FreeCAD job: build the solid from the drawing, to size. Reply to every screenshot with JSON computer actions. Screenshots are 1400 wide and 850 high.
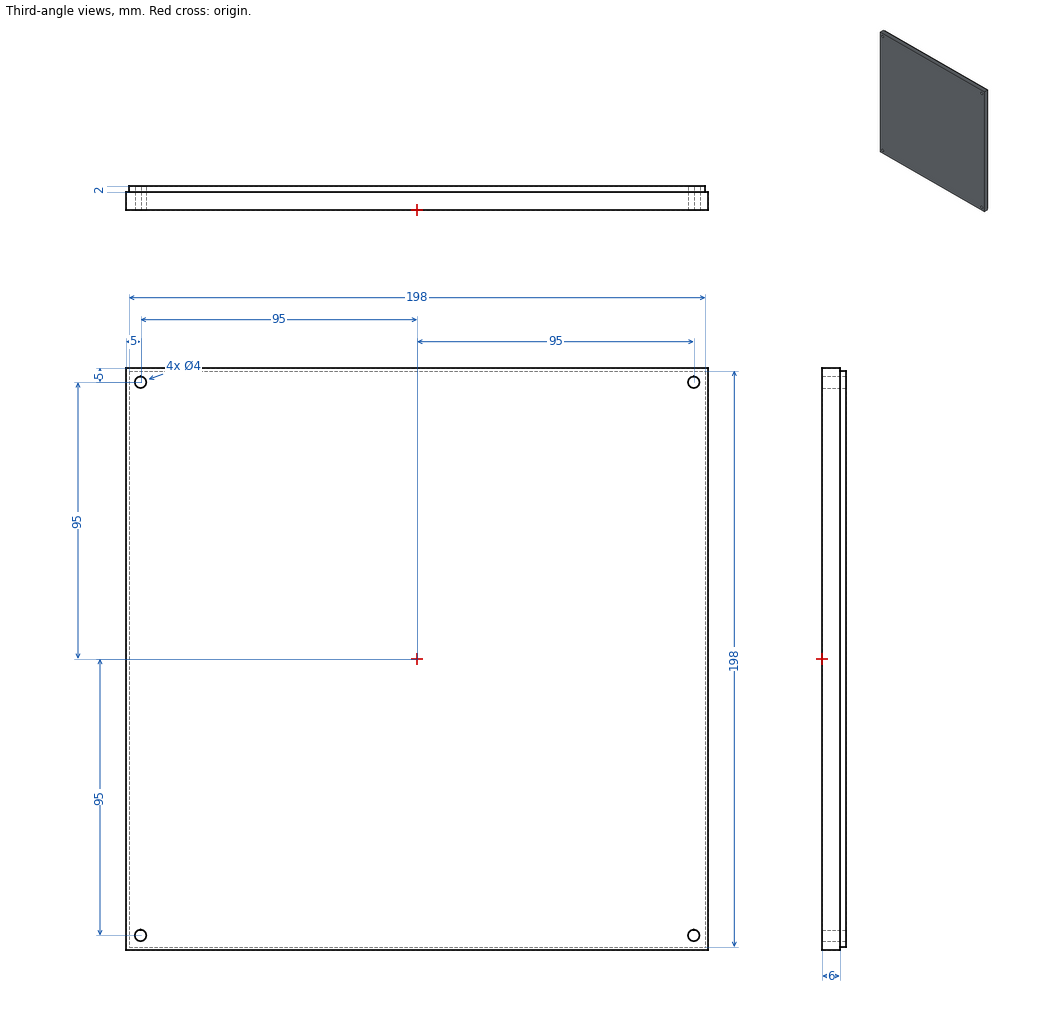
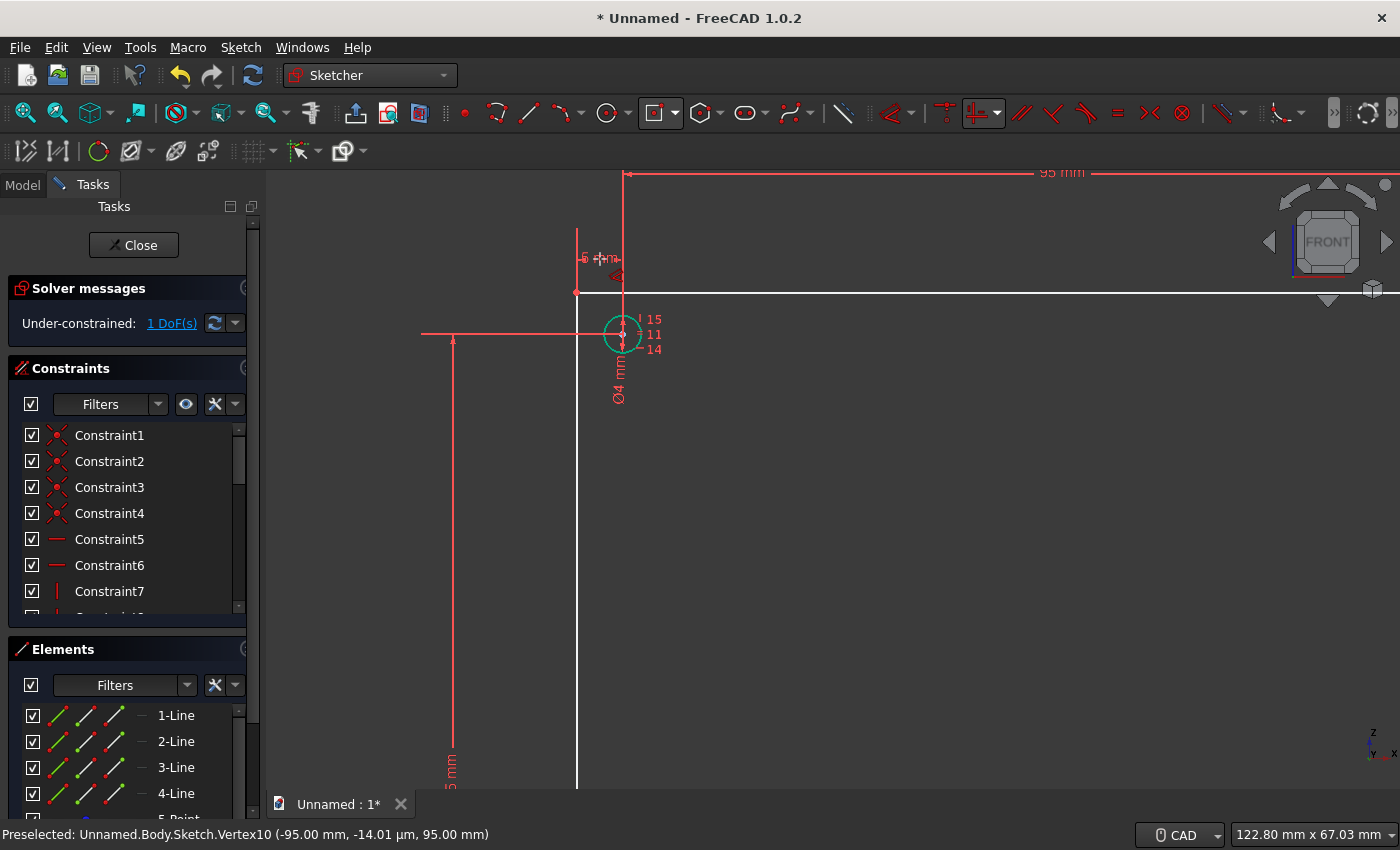
{"action": "left_click", "coordinate": [577, 293]}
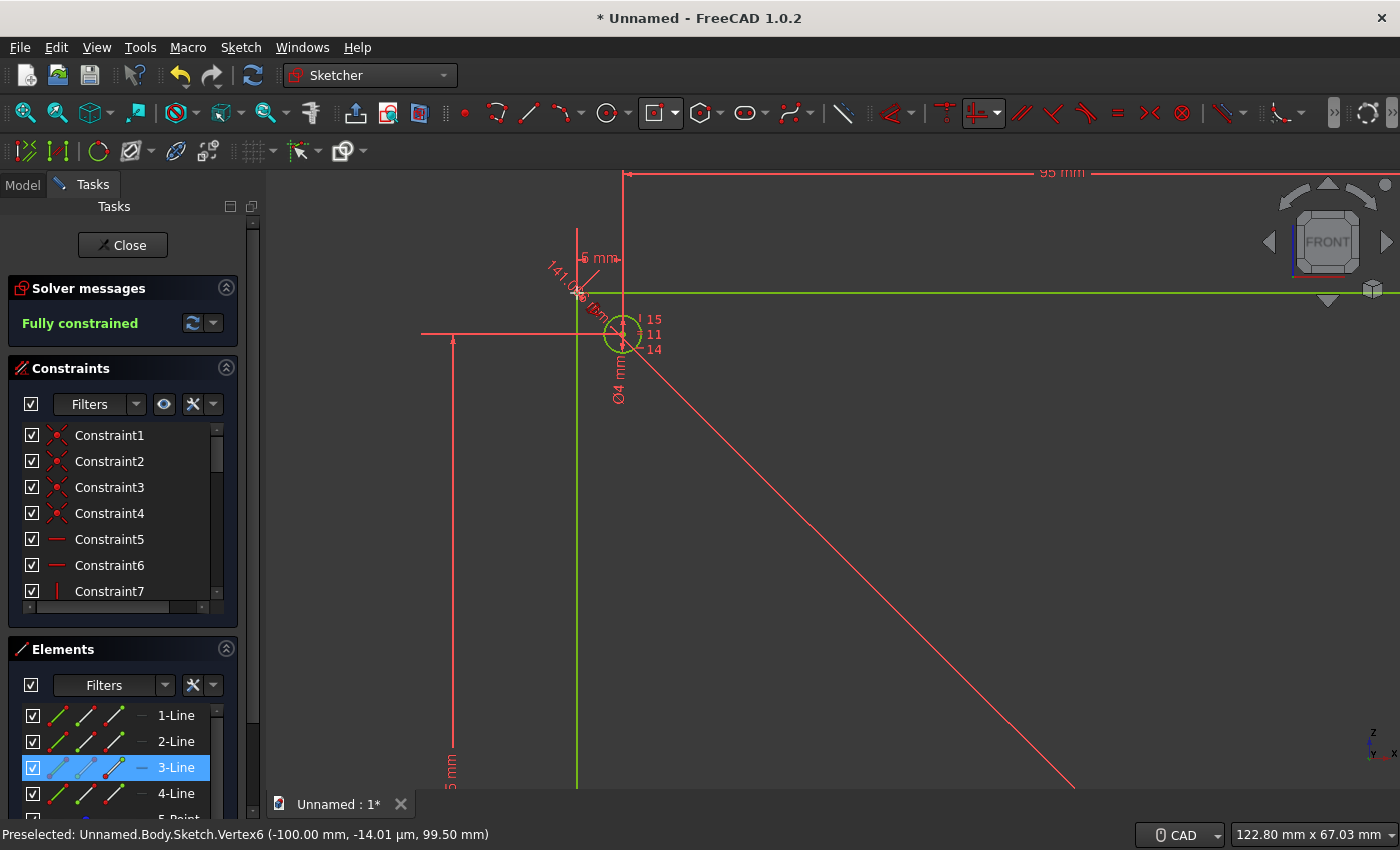
{"action": "left_click", "coordinate": [623, 334]}
{"action": "left_click", "coordinate": [543, 314]}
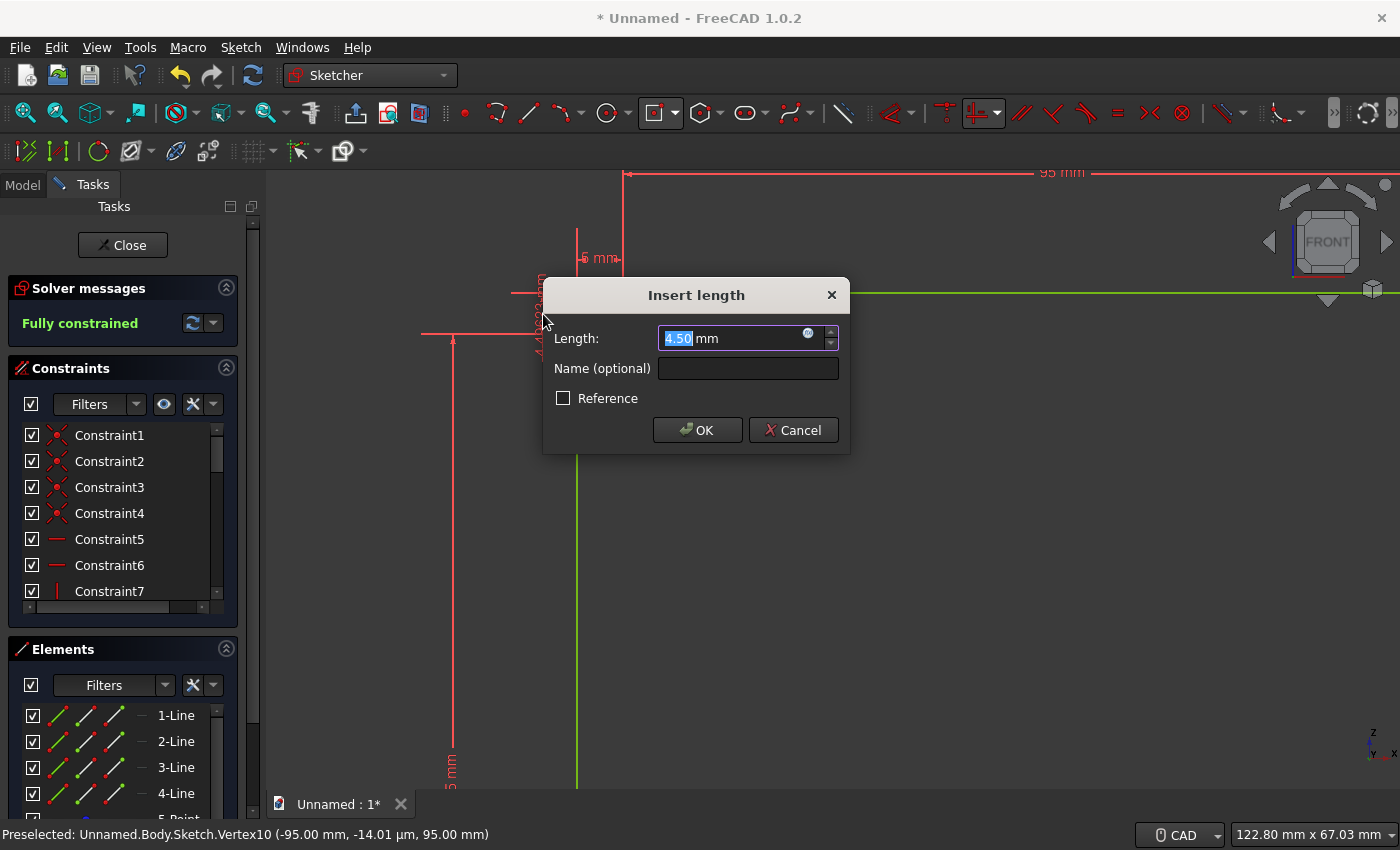
{"action": "type", "text": "5"}
{"action": "key", "text": "Return"}
{"action": "key", "text": "Escape"}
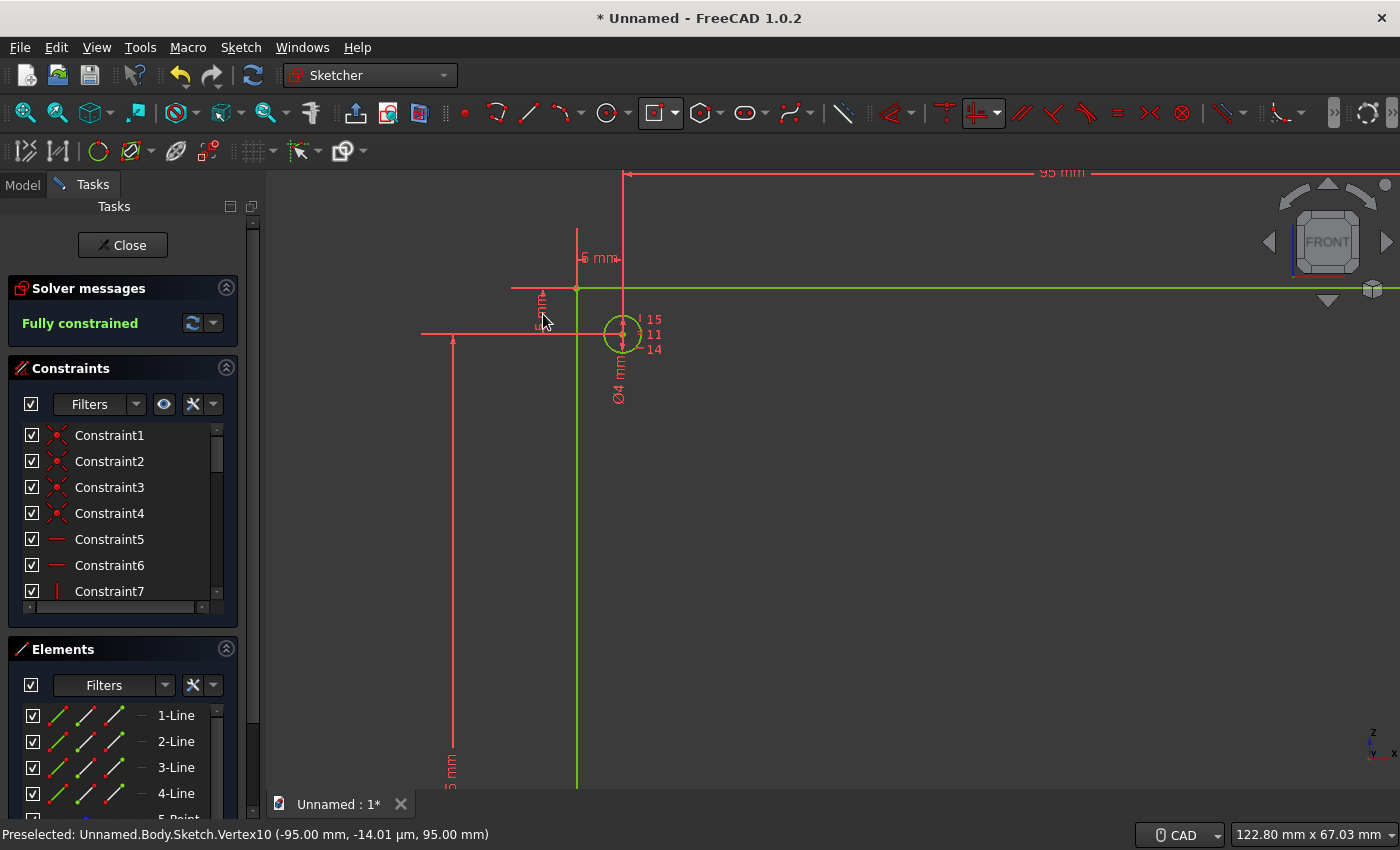
{"action": "left_click", "coordinate": [123, 245]}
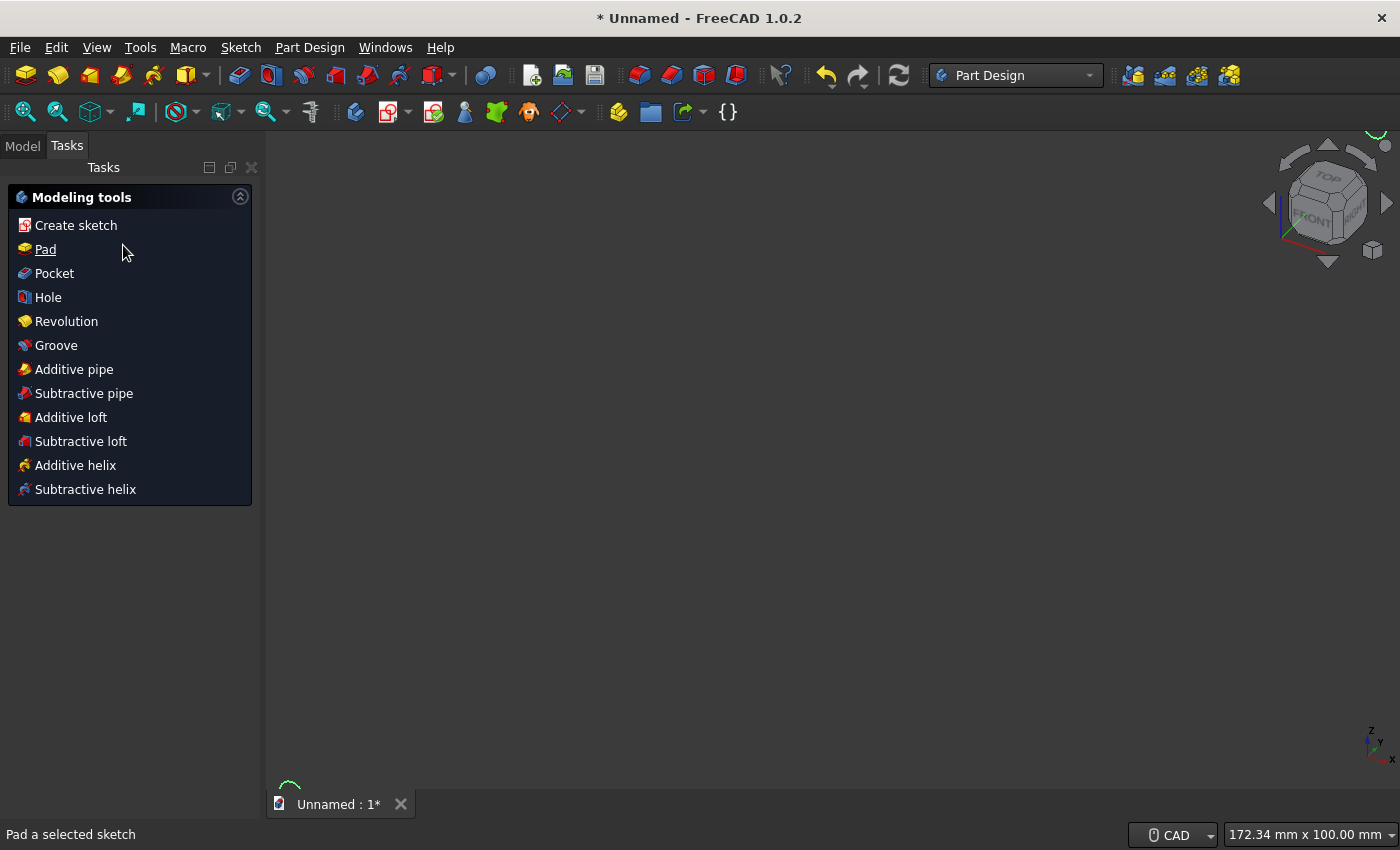
{"action": "left_click", "coordinate": [26, 76]}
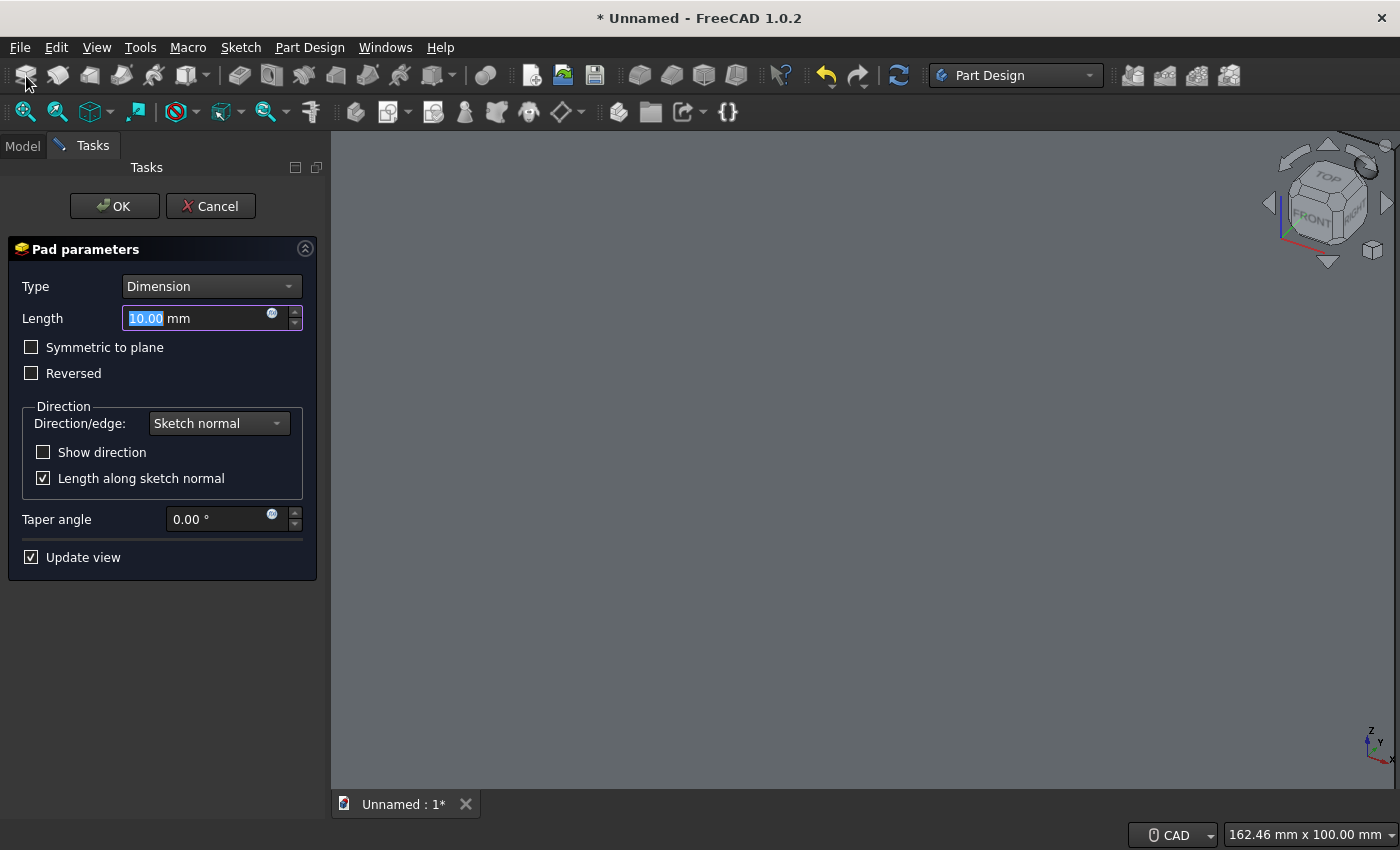
{"action": "type", "text": "6"}
{"action": "key", "text": "Tab"}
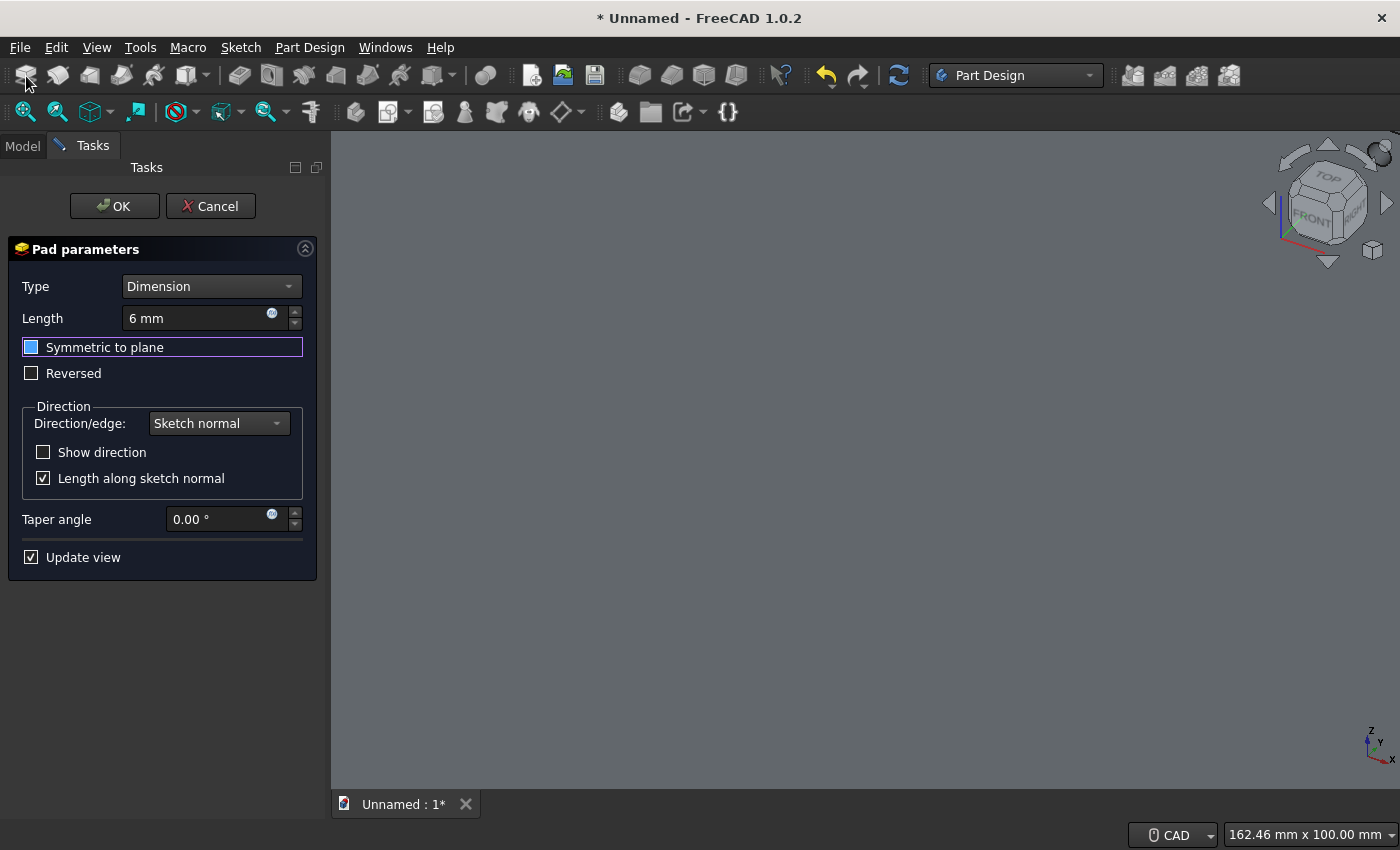
{"action": "left_click", "coordinate": [30, 373]}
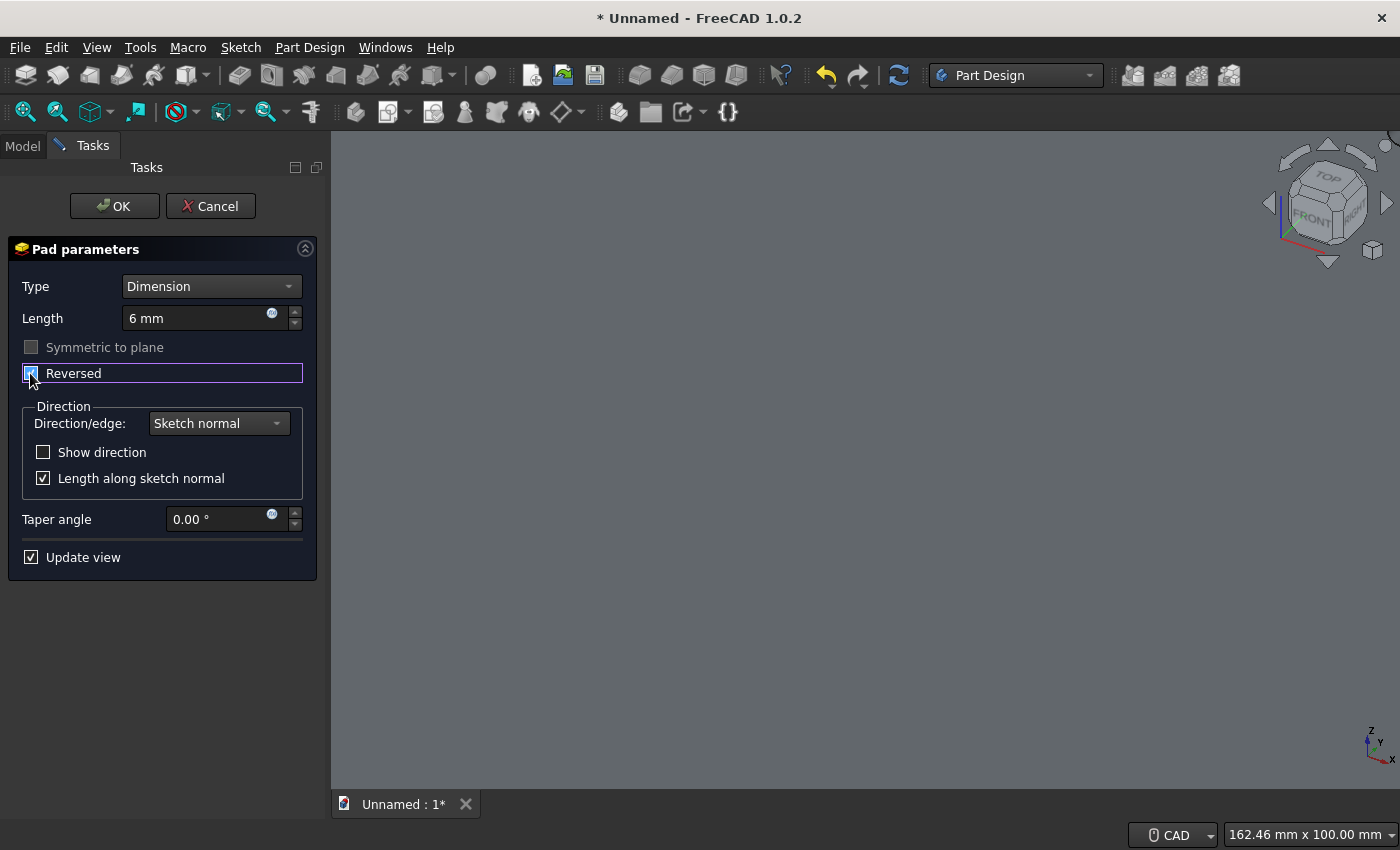
{"action": "left_click", "coordinate": [115, 206]}